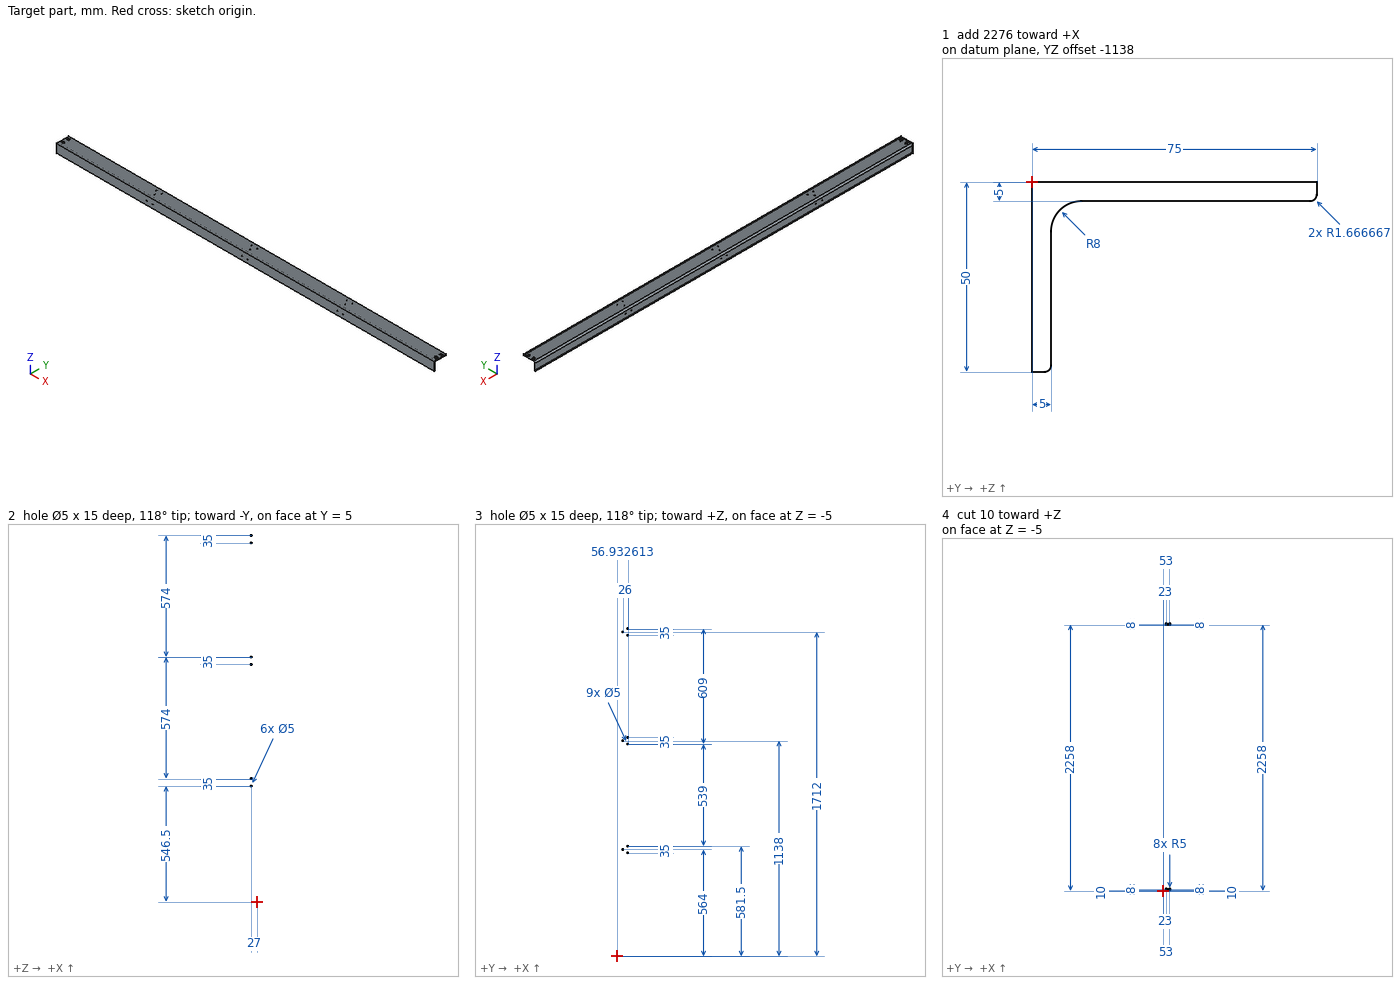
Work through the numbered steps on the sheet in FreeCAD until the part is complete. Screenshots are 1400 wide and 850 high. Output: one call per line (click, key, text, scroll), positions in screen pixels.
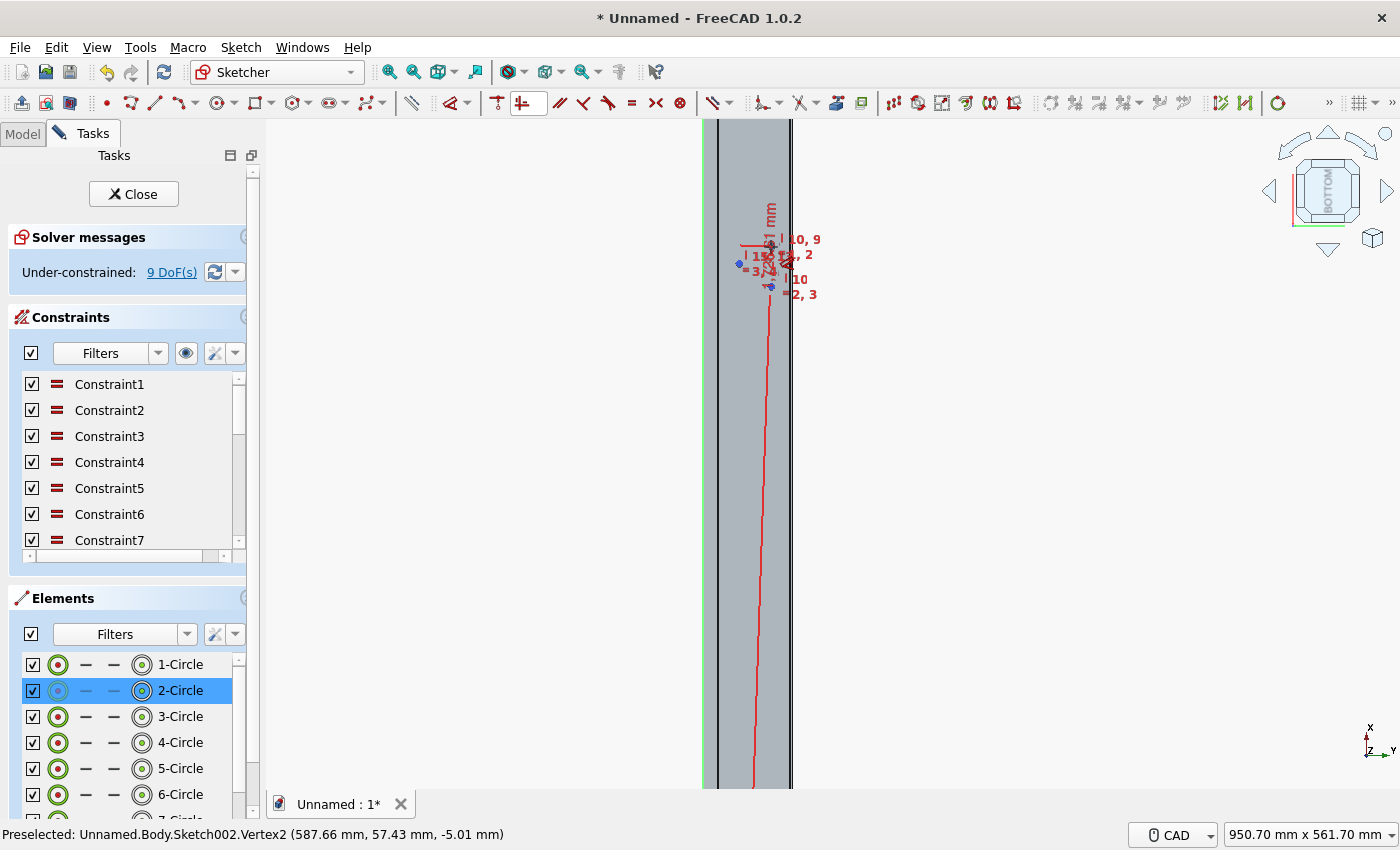
click(771, 287)
click(805, 267)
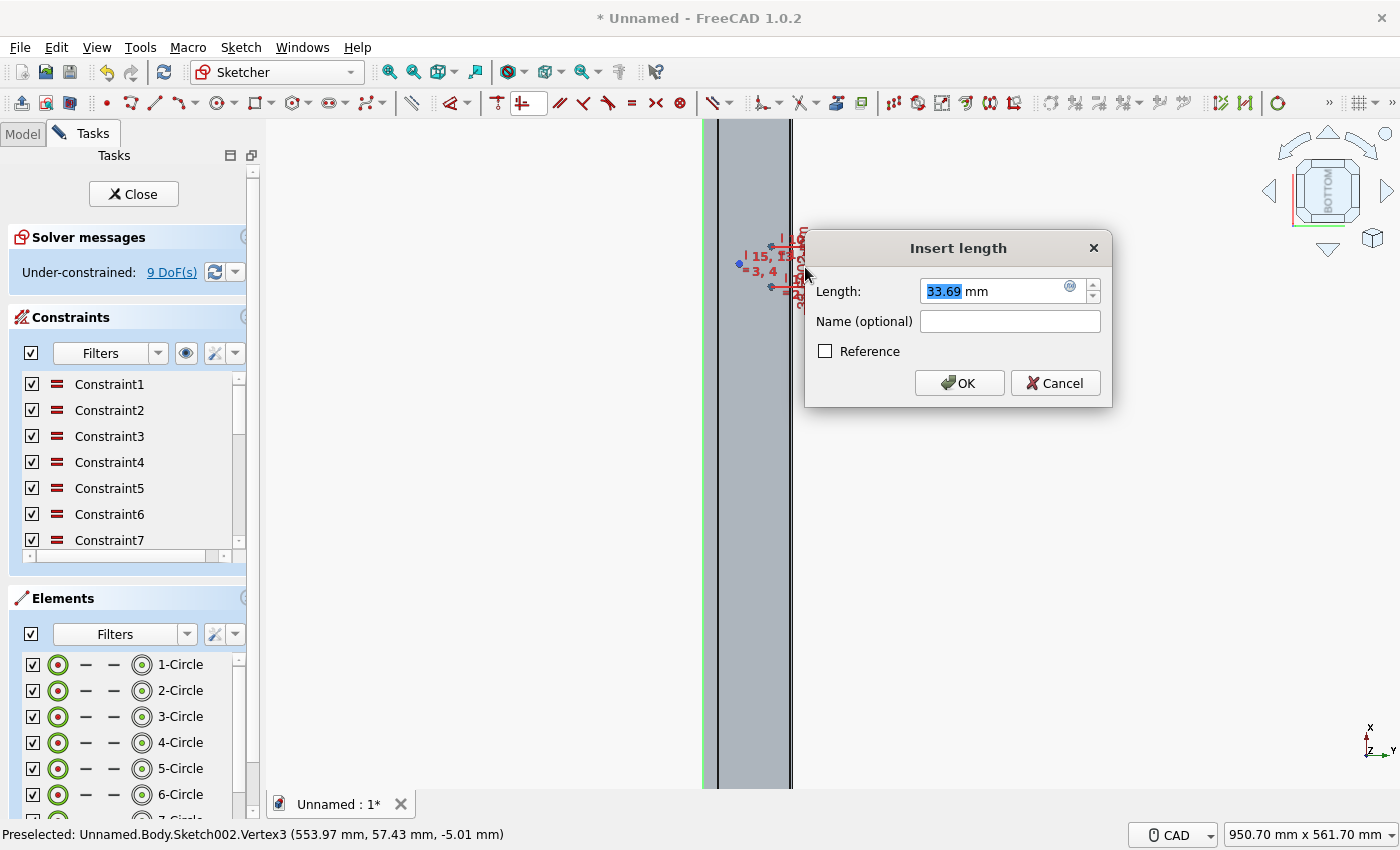
text(35)
key(Return)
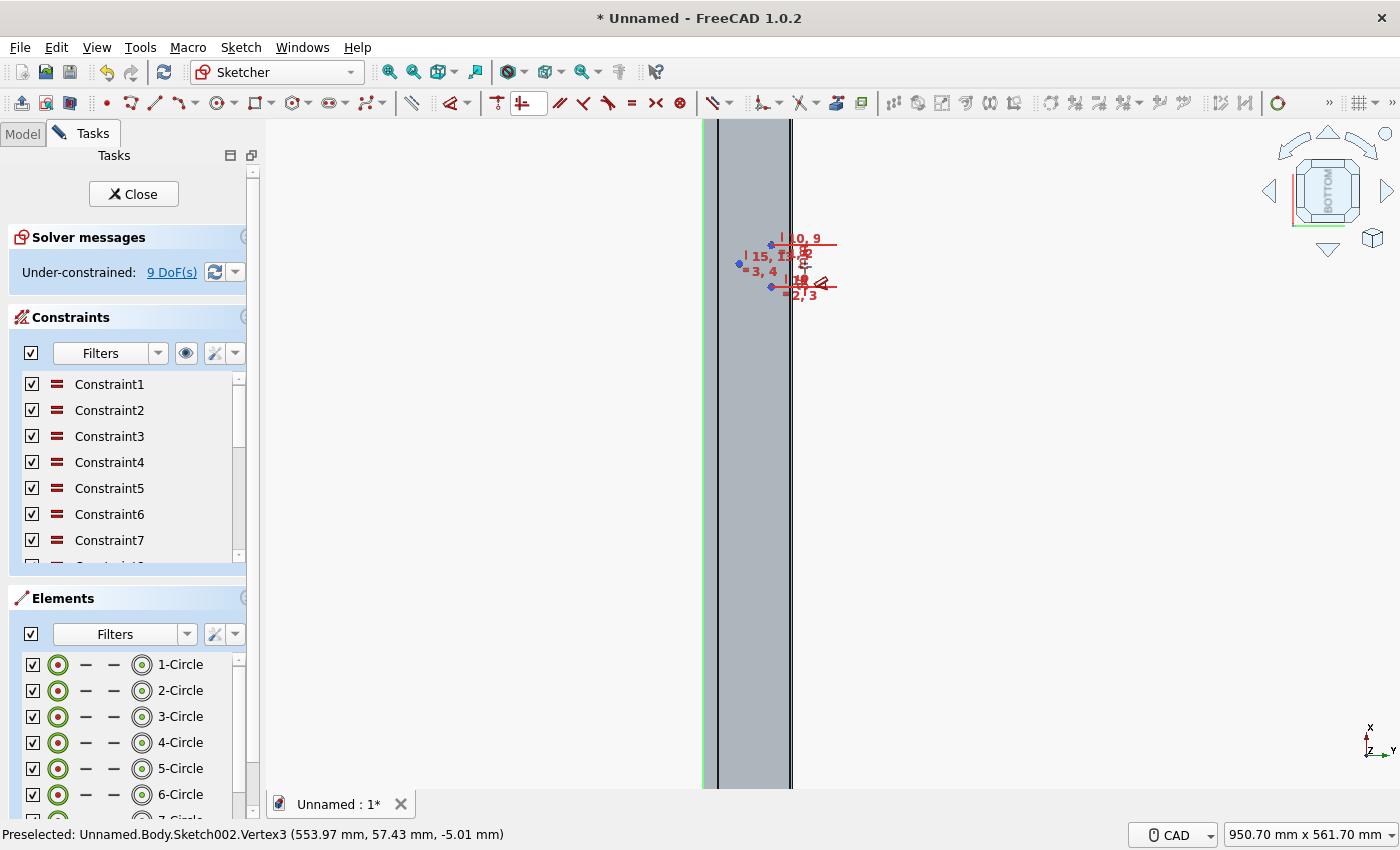
scroll(771, 245, up, 2)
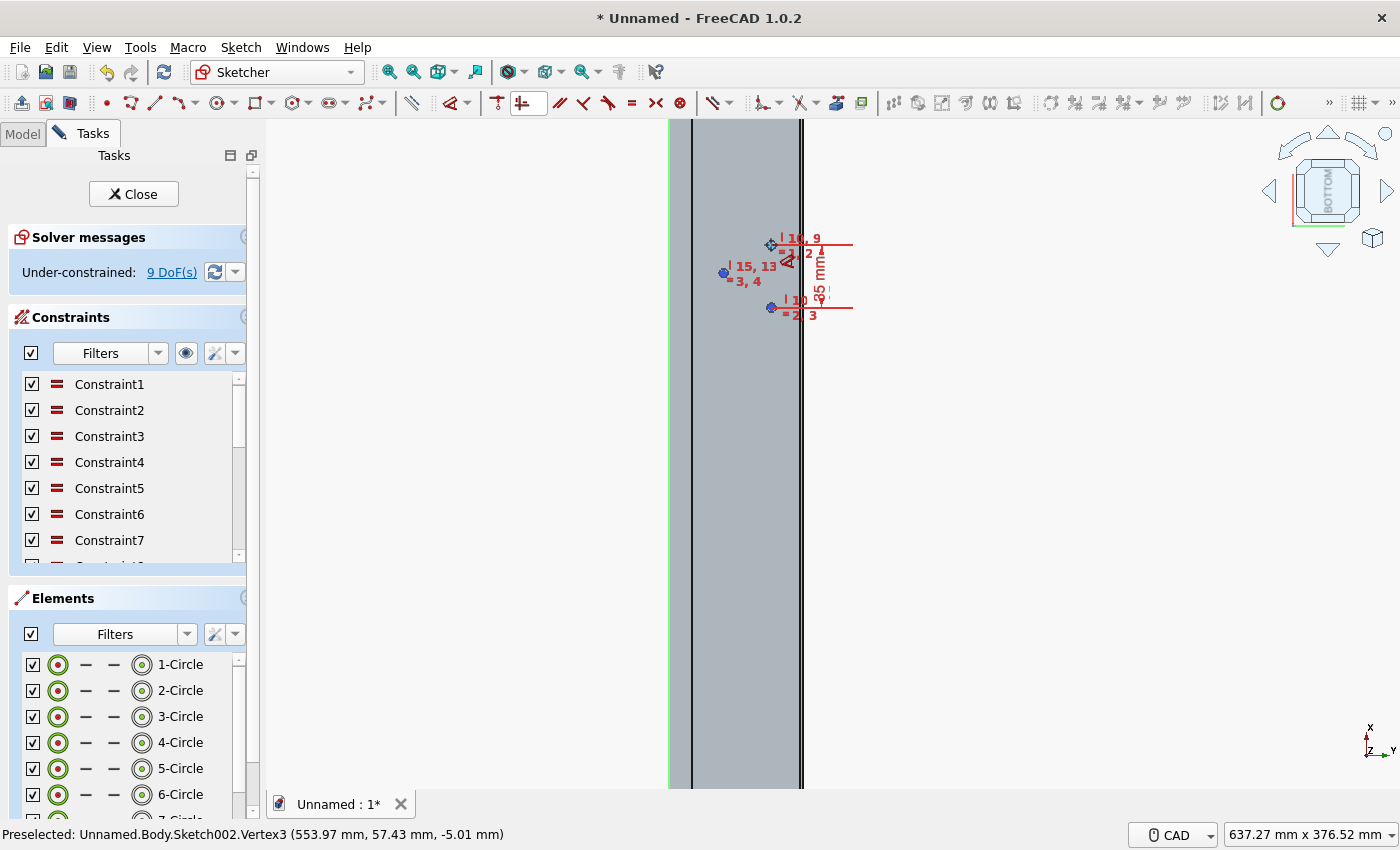
click(771, 245)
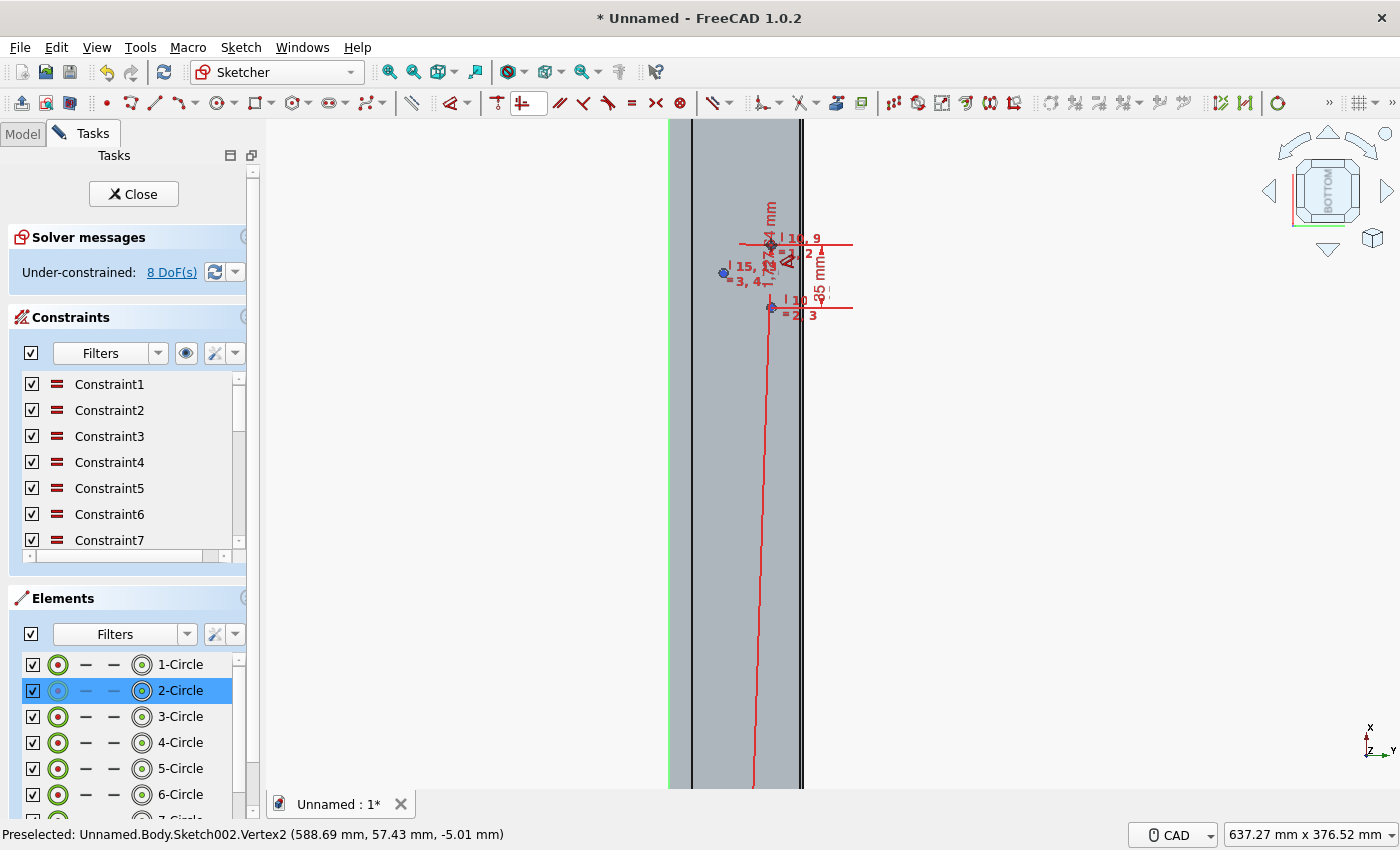
click(724, 273)
click(748, 211)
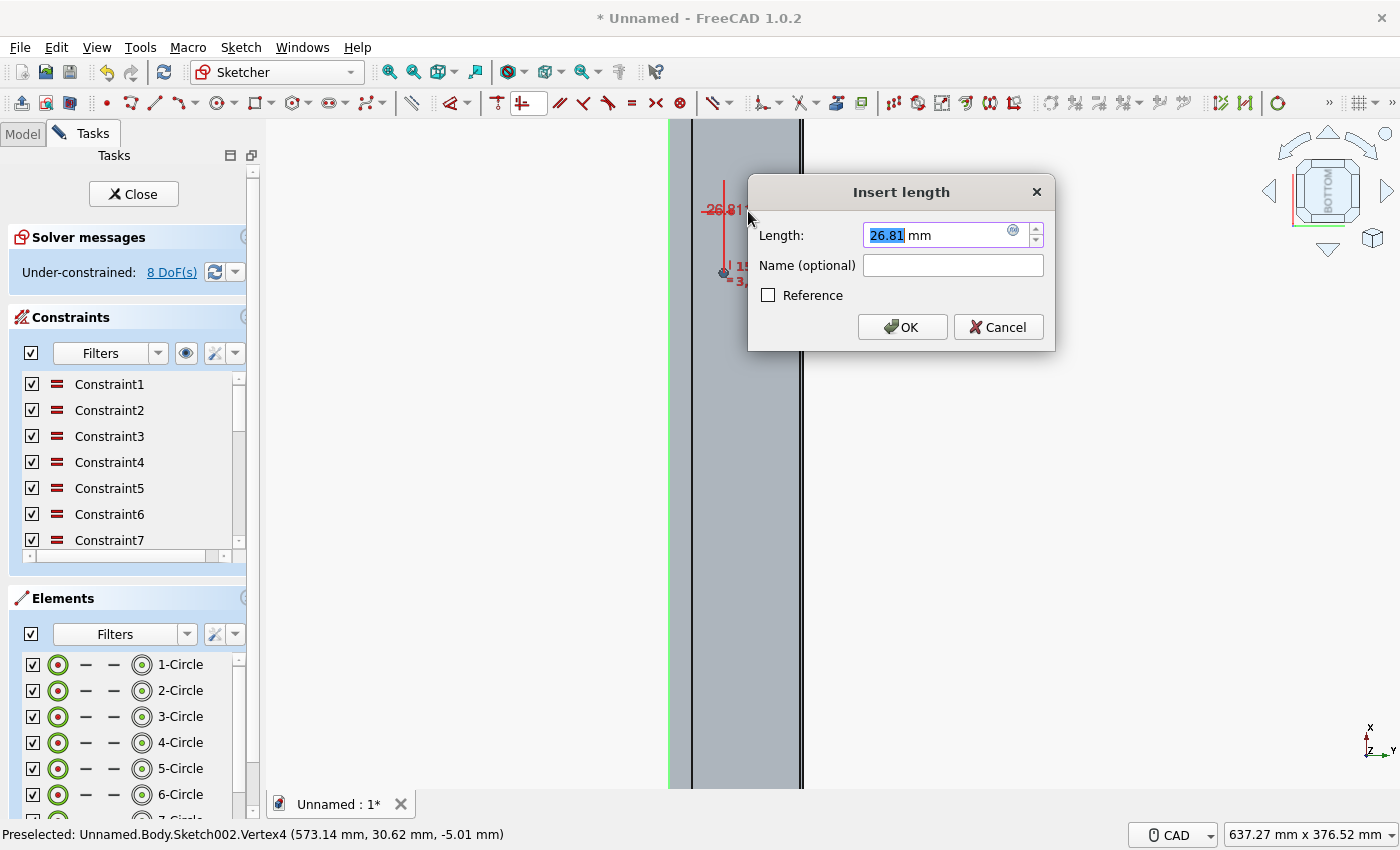
text(26)
key(Return)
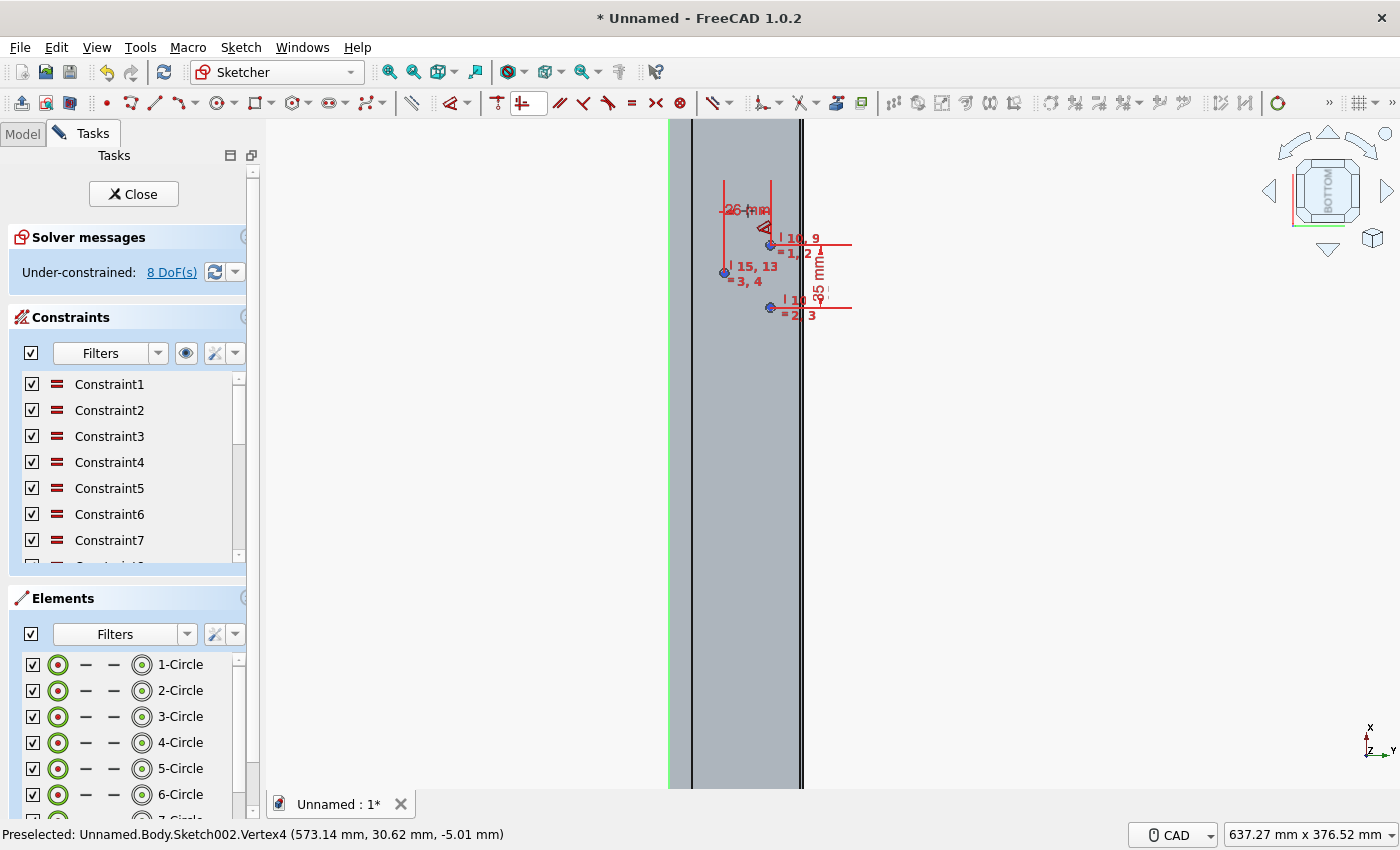
scroll(771, 247, down, 10)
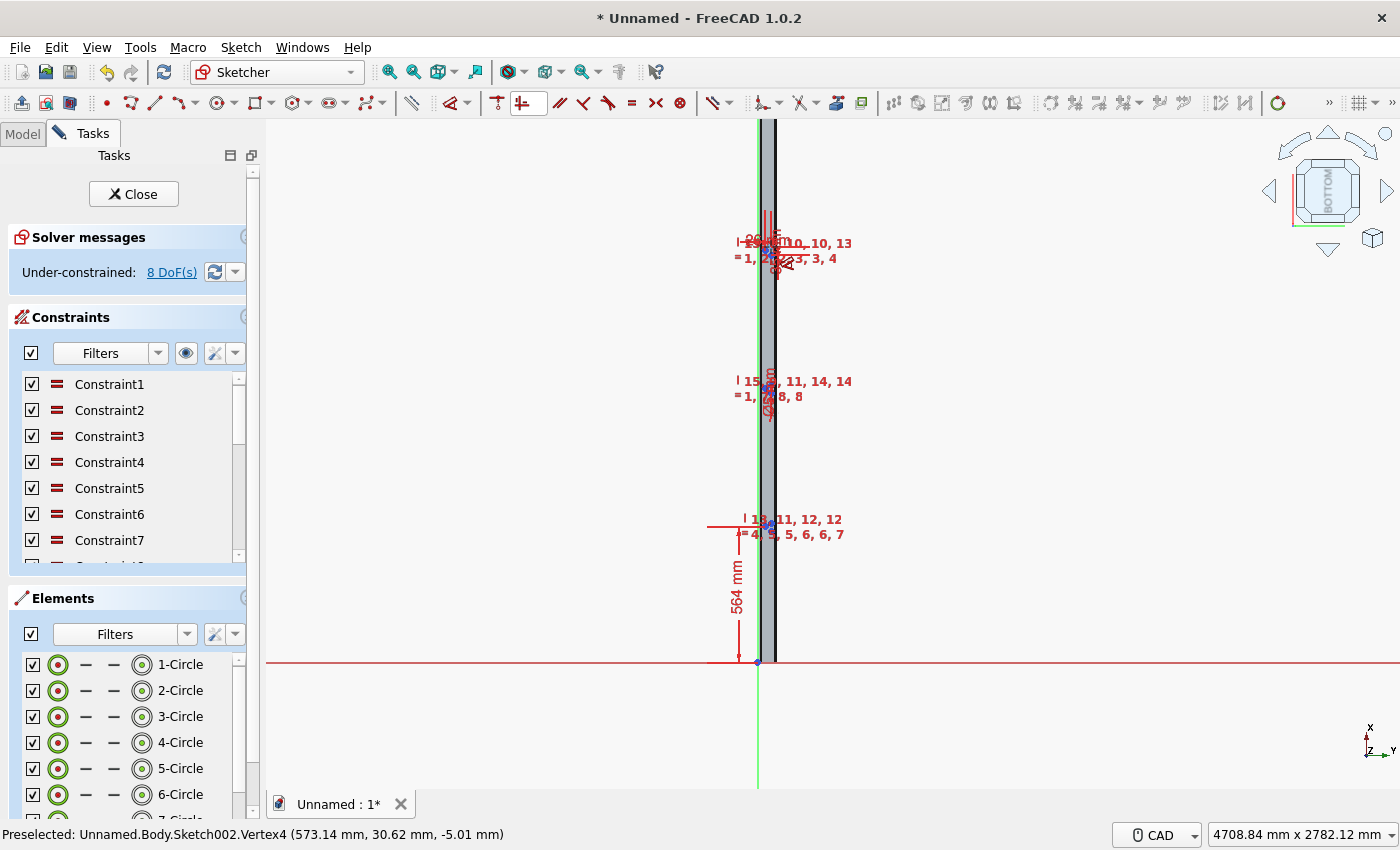
scroll(771, 523, up, 8)